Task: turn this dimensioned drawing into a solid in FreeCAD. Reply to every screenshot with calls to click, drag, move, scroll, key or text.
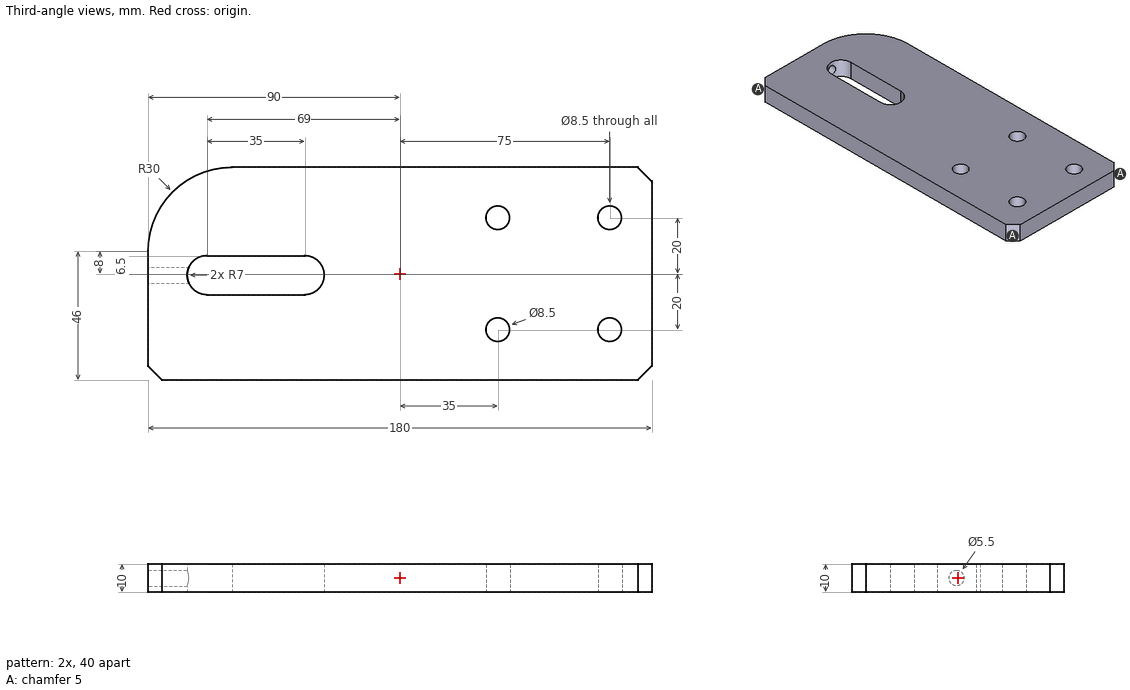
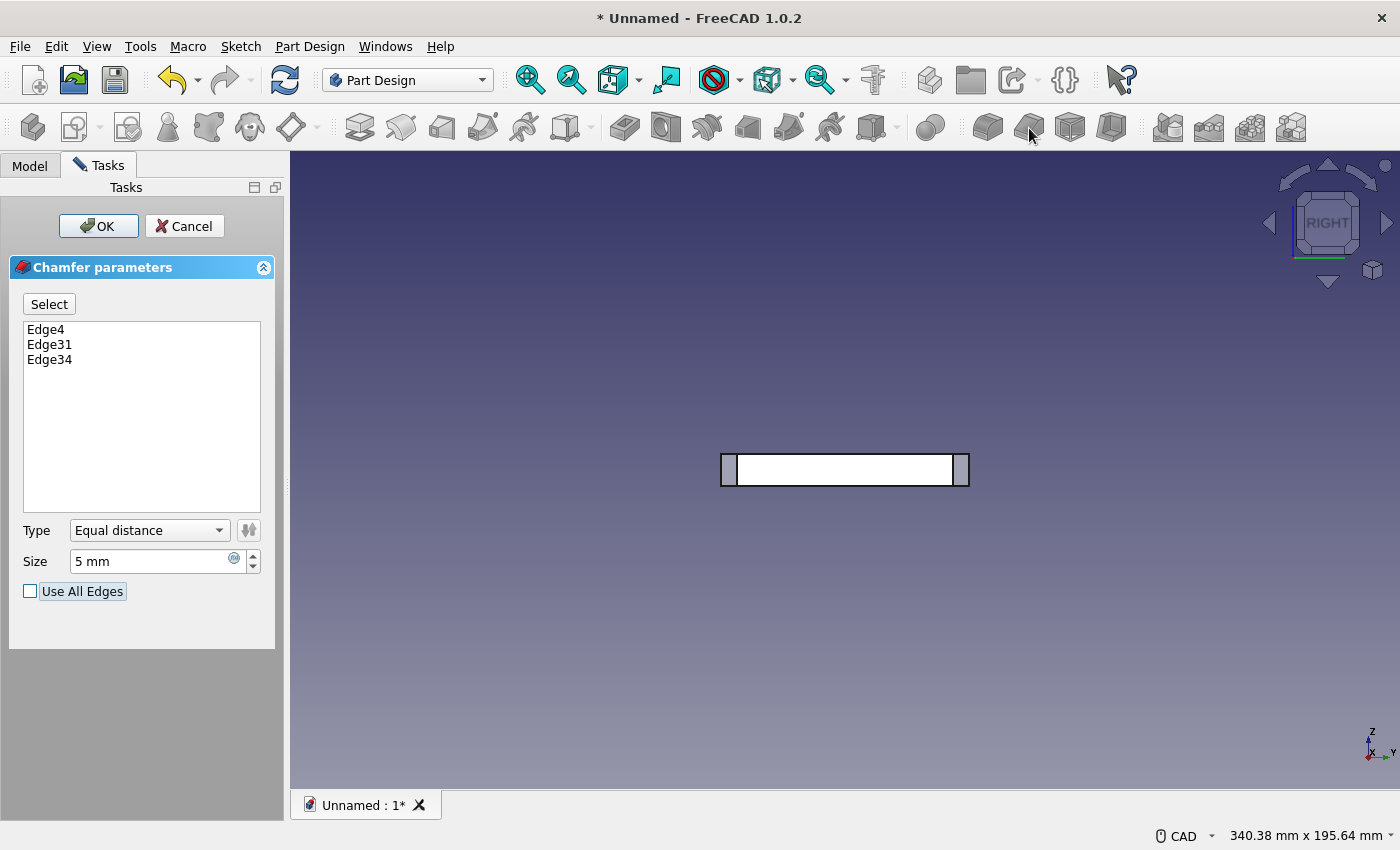
click(99, 226)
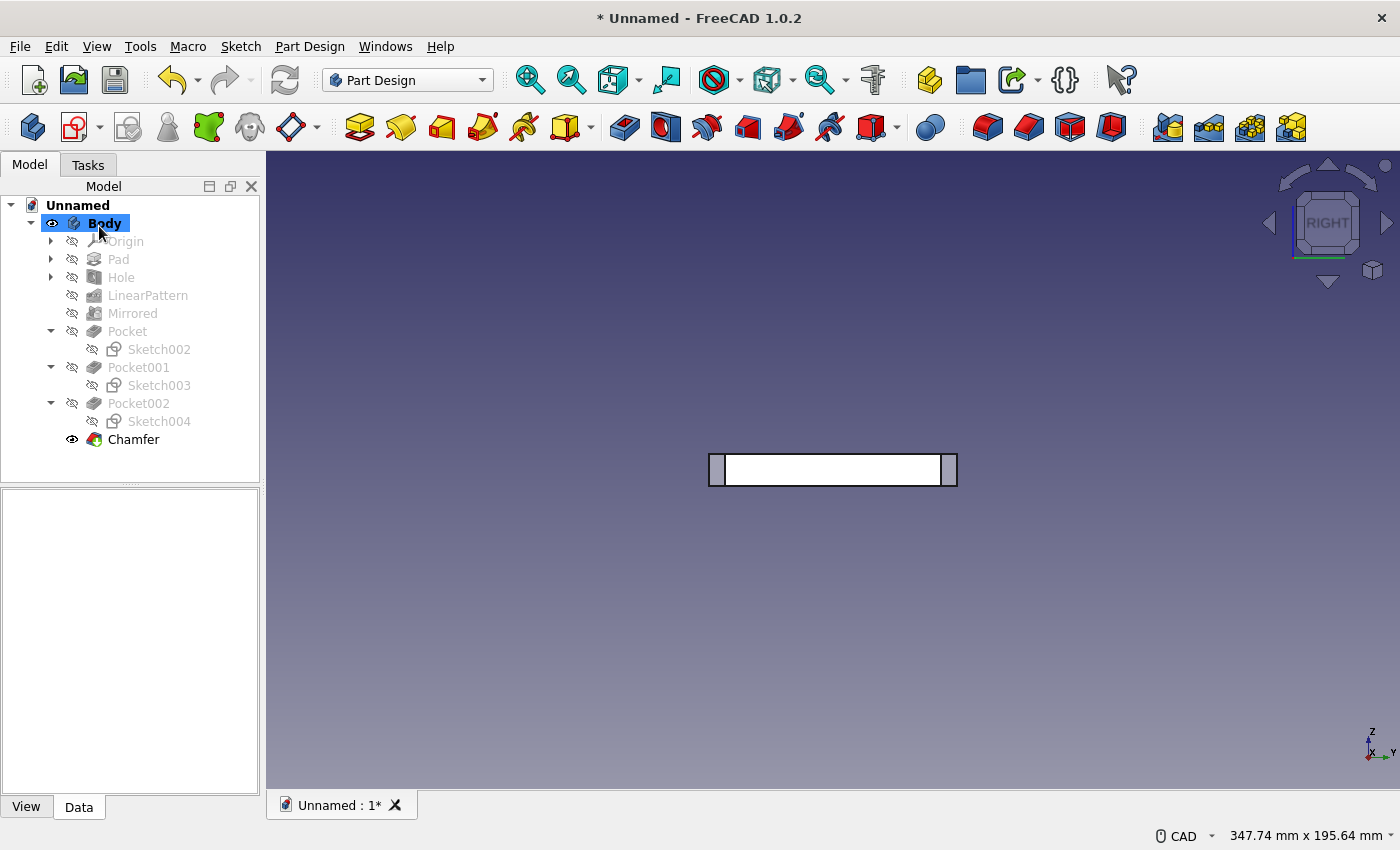
key(0)